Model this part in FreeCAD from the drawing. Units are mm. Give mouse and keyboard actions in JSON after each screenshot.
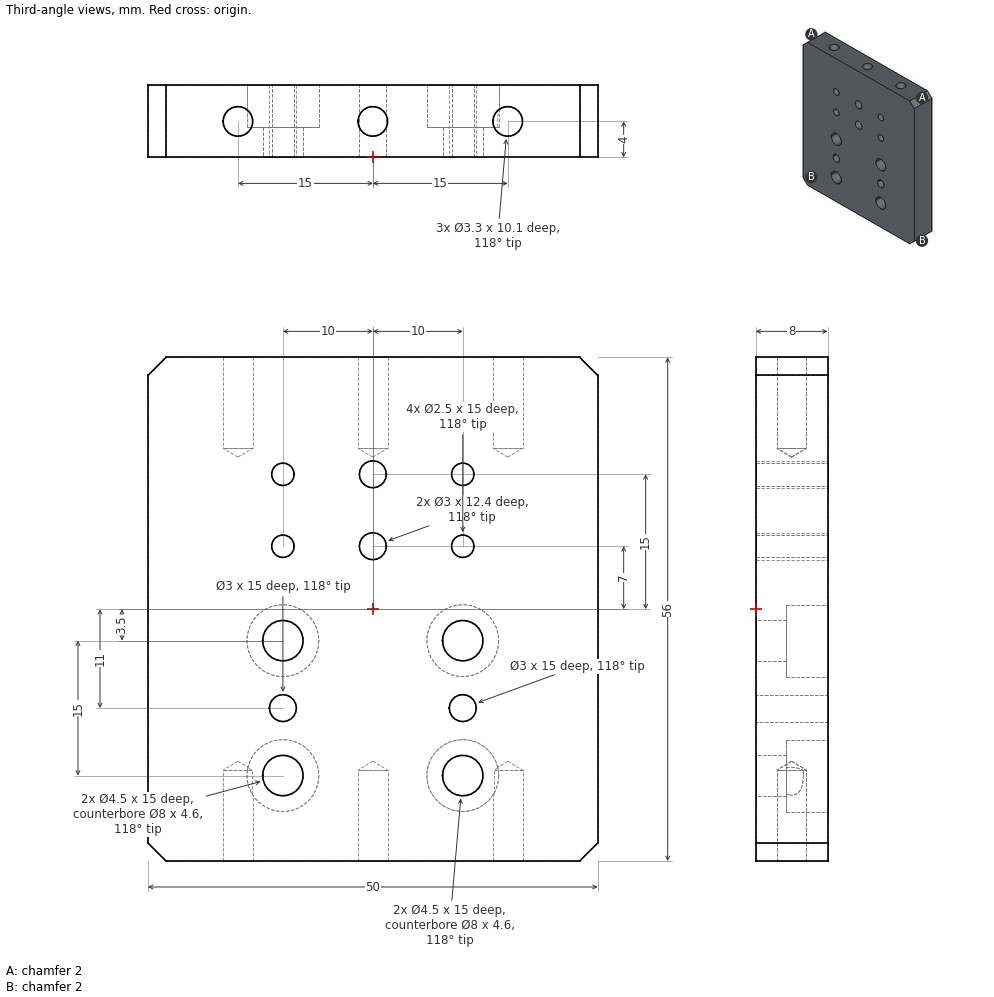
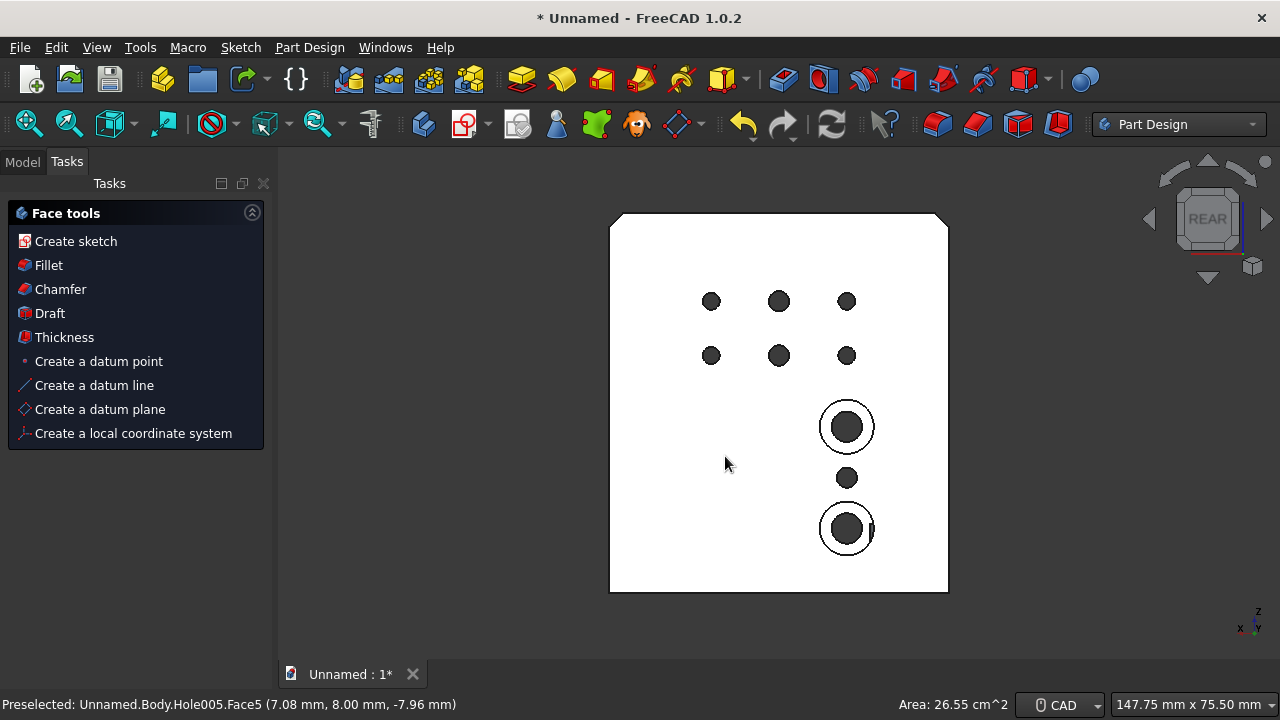
{"action": "left_click", "coordinate": [464, 124]}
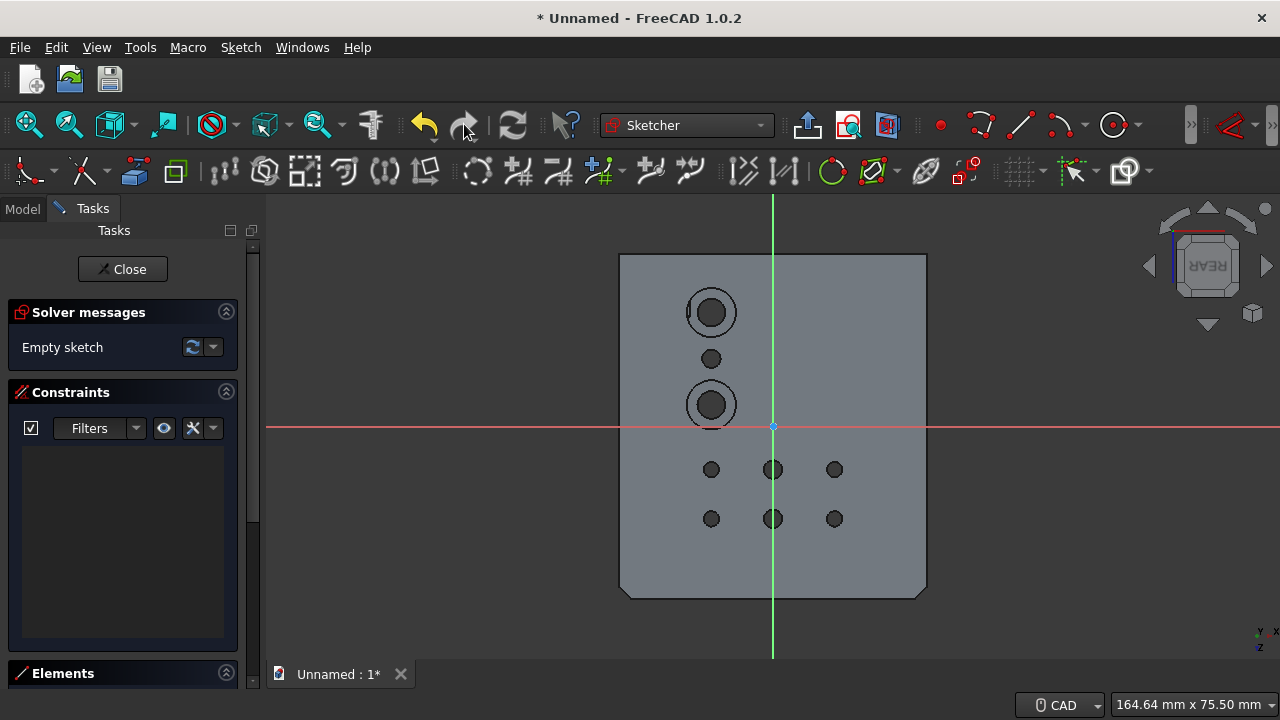
{"action": "scroll", "coordinate": [897, 310], "scroll_direction": "up", "scroll_amount": 4}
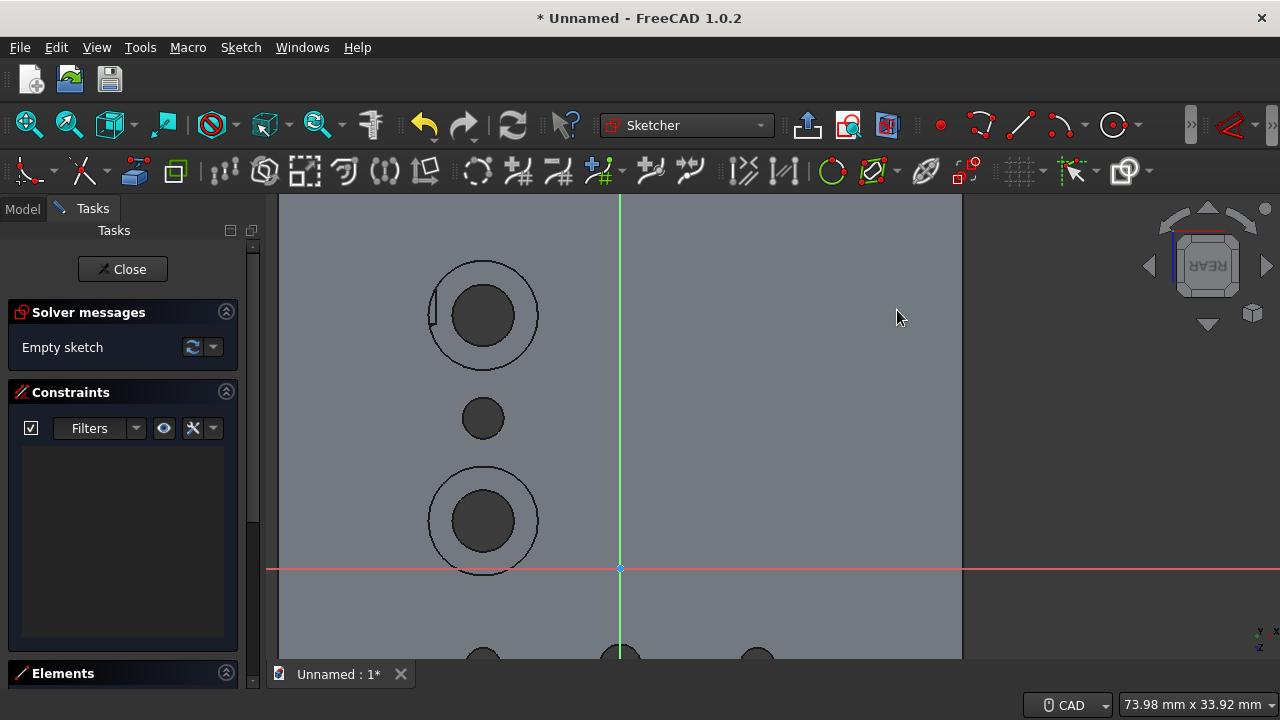
{"action": "key", "text": "g c"}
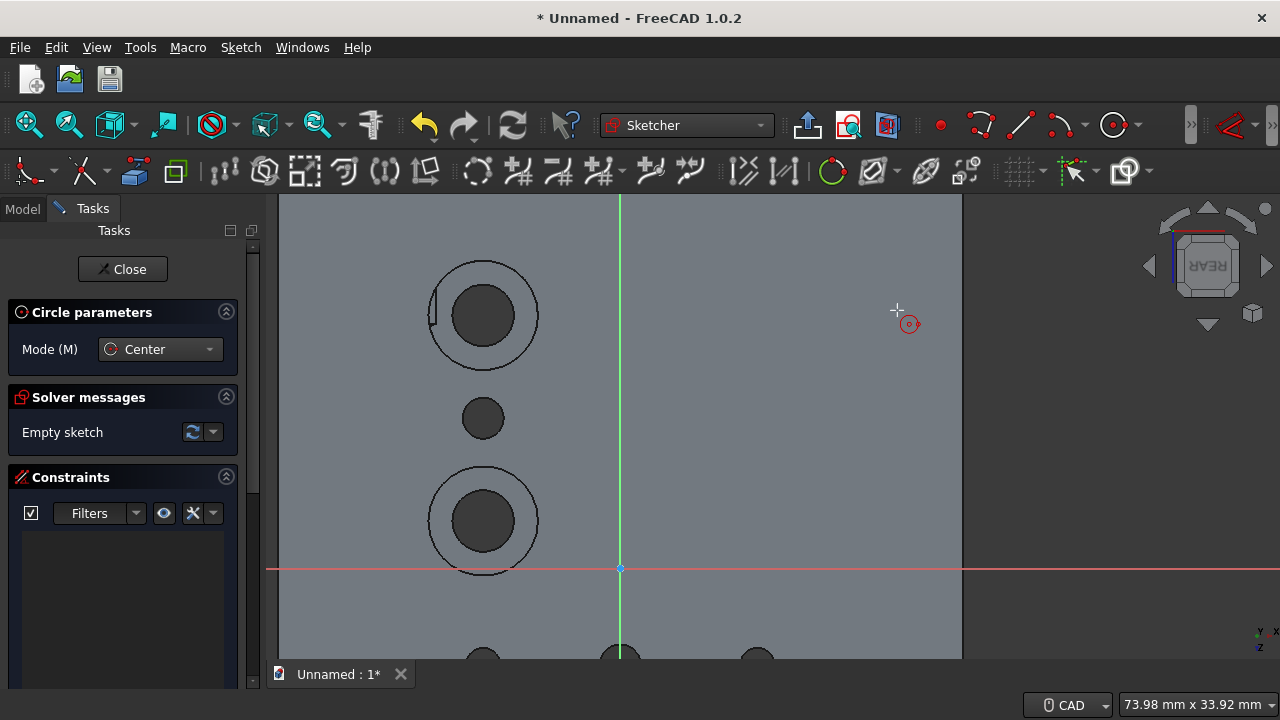
{"action": "left_click", "coordinate": [757, 315]}
{"action": "mouse_move", "coordinate": [779, 294]}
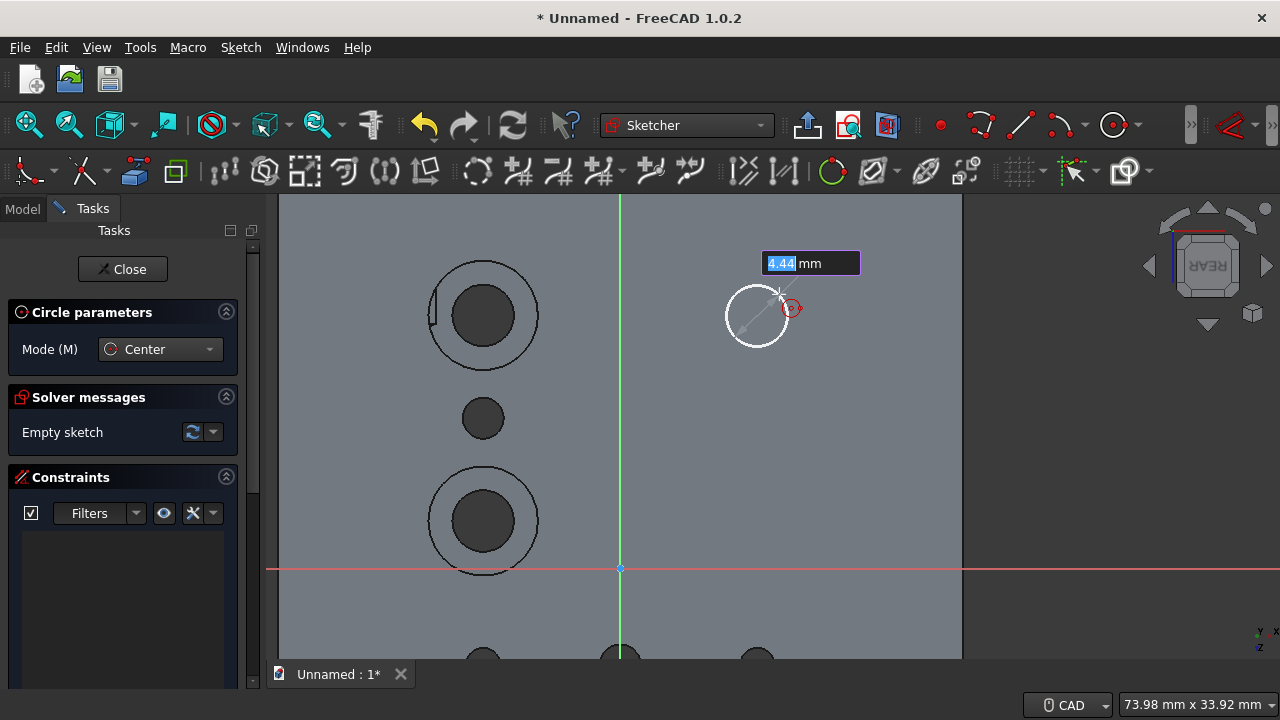
{"action": "type", "text": "4.5"}
{"action": "key", "text": "Return"}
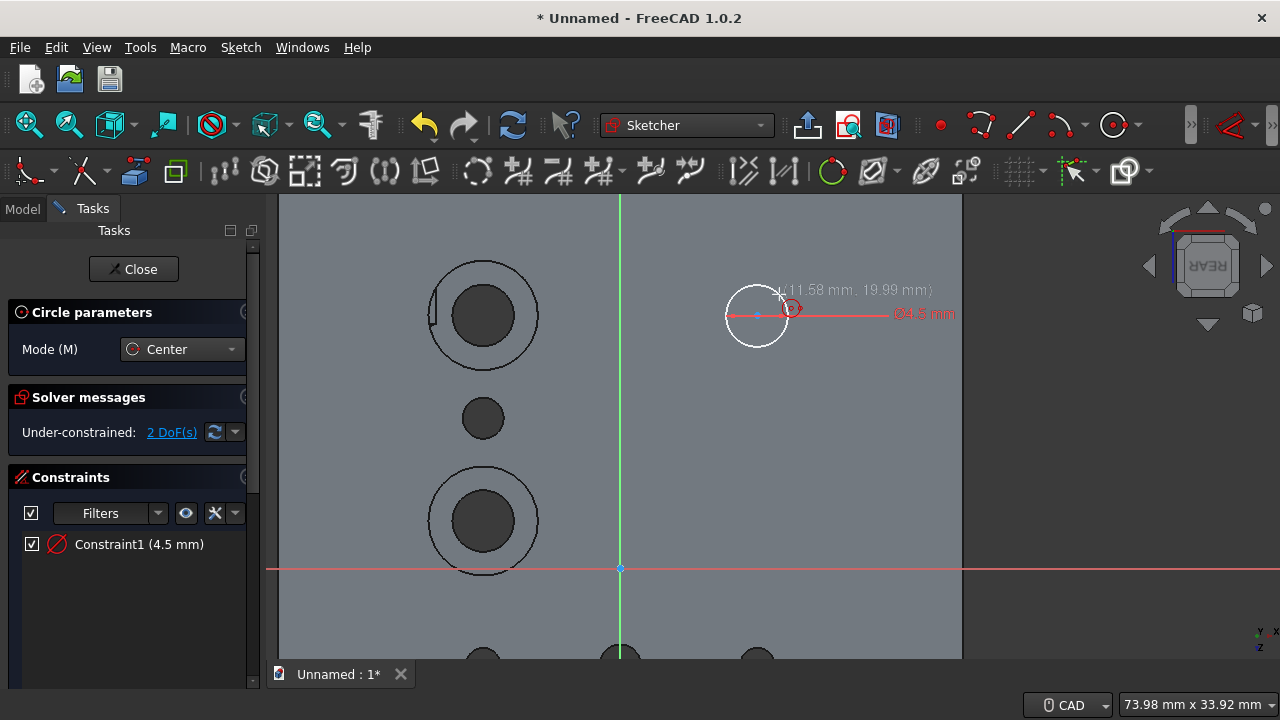
{"action": "left_click", "coordinate": [757, 521]}
{"action": "mouse_move", "coordinate": [779, 499]}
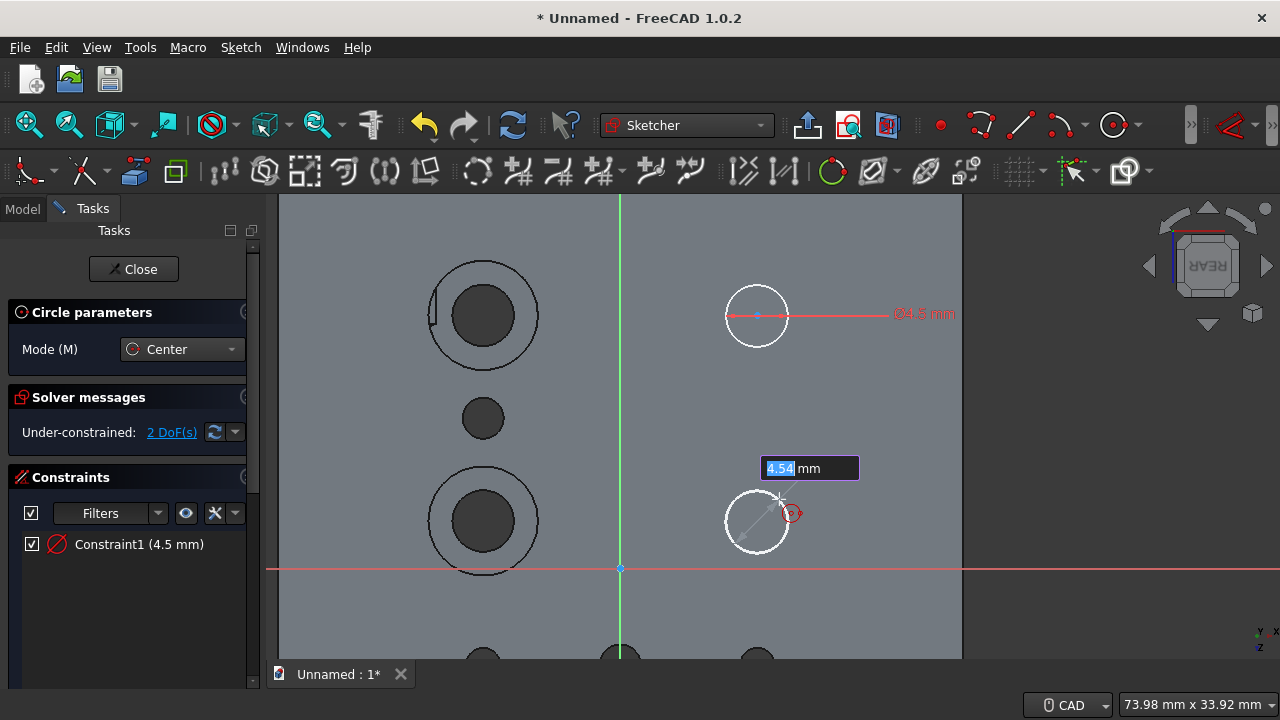
{"action": "type", "text": "4.5"}
{"action": "key", "text": "Return"}
{"action": "key", "text": "Escape"}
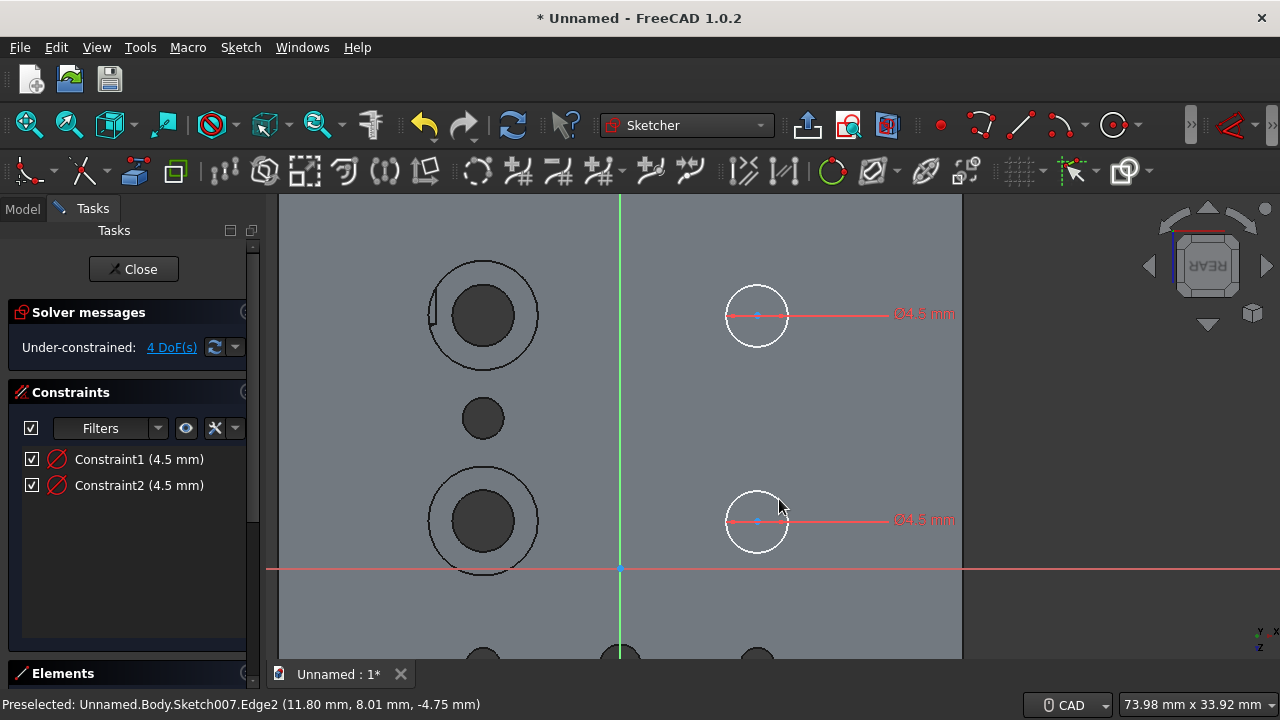
{"action": "left_click", "coordinate": [757, 316]}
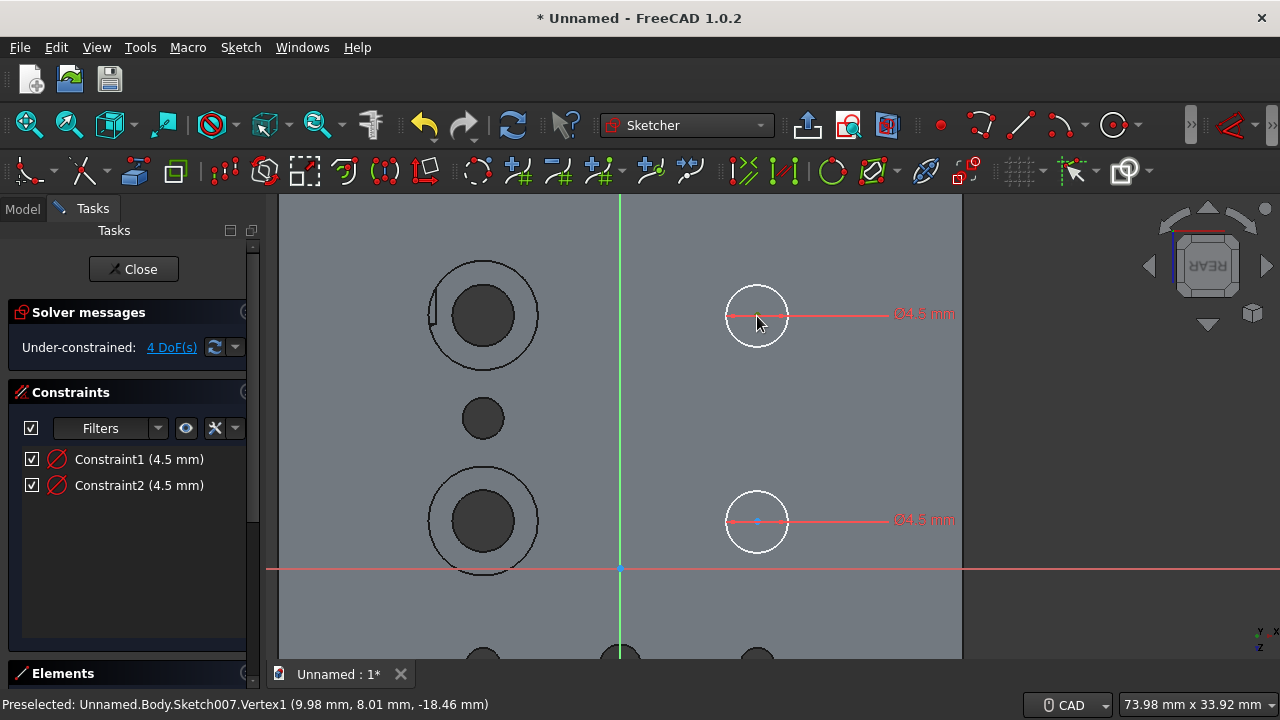
{"action": "left_click", "coordinate": [757, 522]}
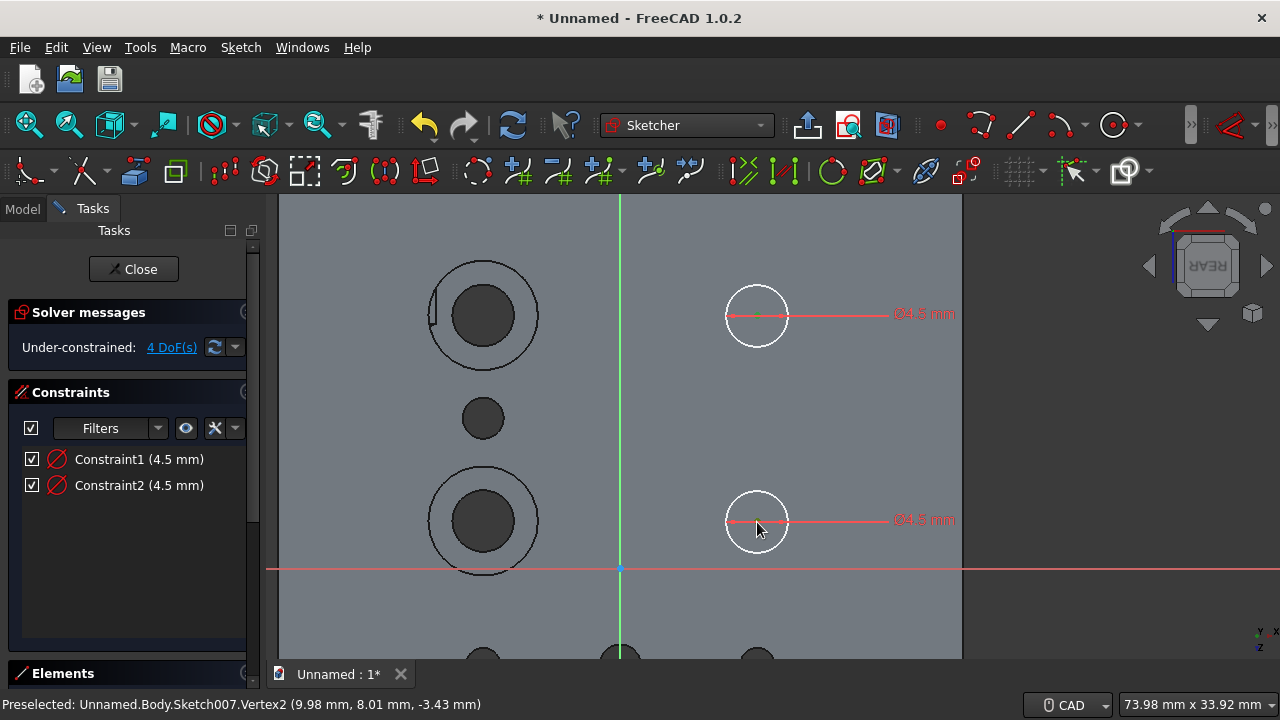
{"action": "key", "text": "v"}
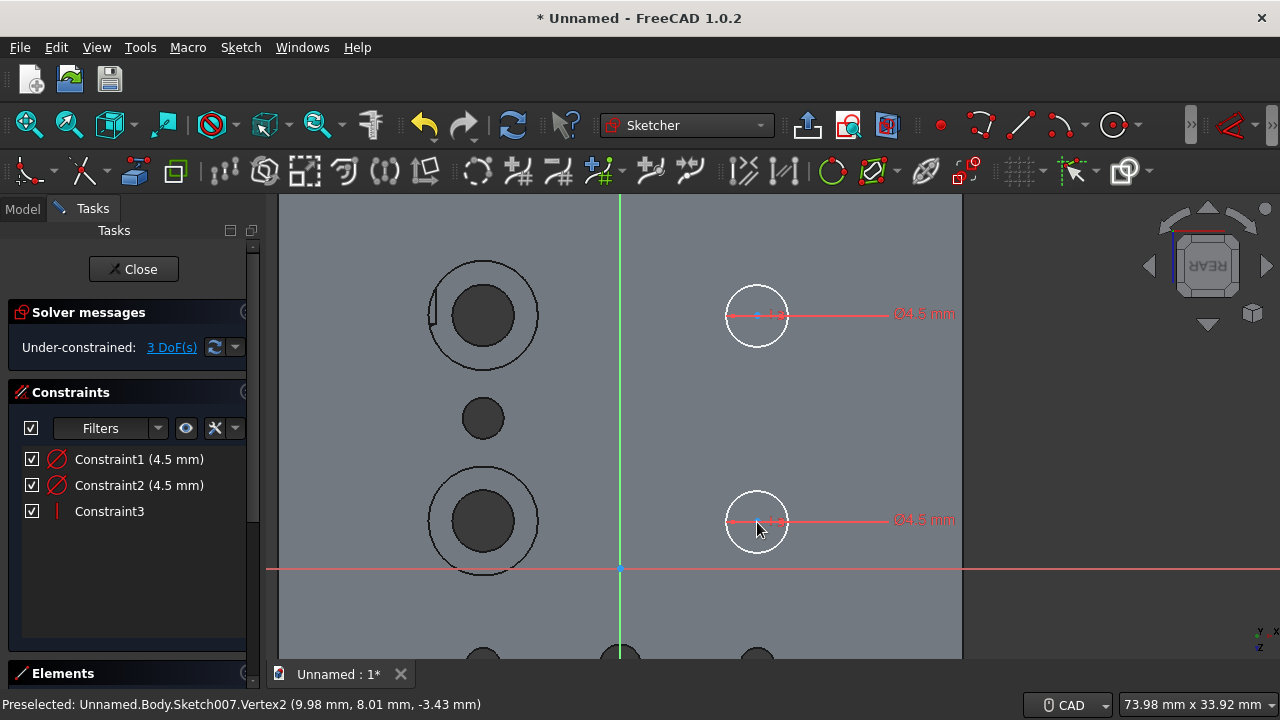
{"action": "left_click", "coordinate": [1230, 126]}